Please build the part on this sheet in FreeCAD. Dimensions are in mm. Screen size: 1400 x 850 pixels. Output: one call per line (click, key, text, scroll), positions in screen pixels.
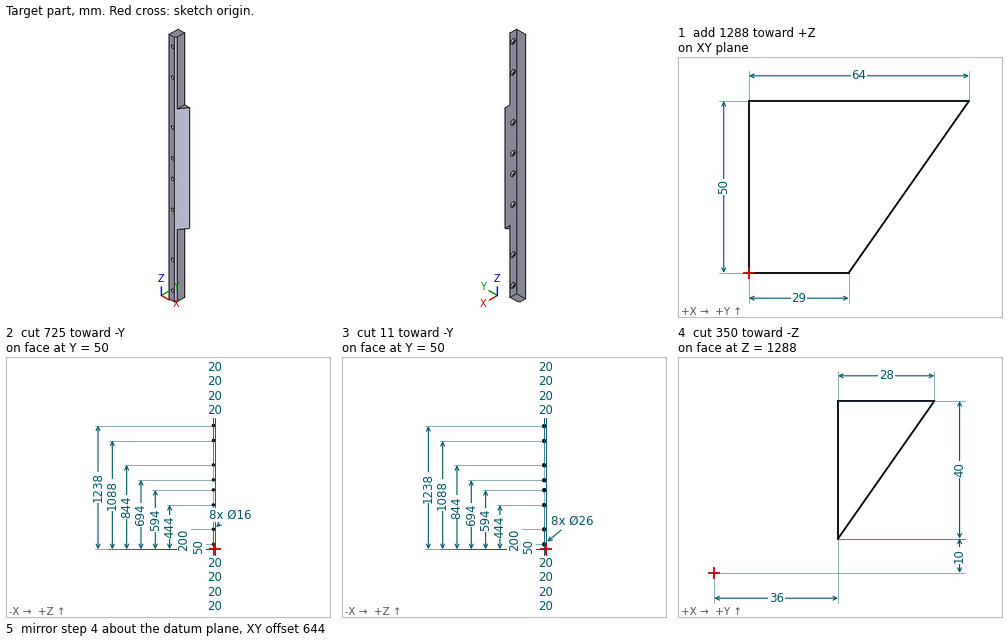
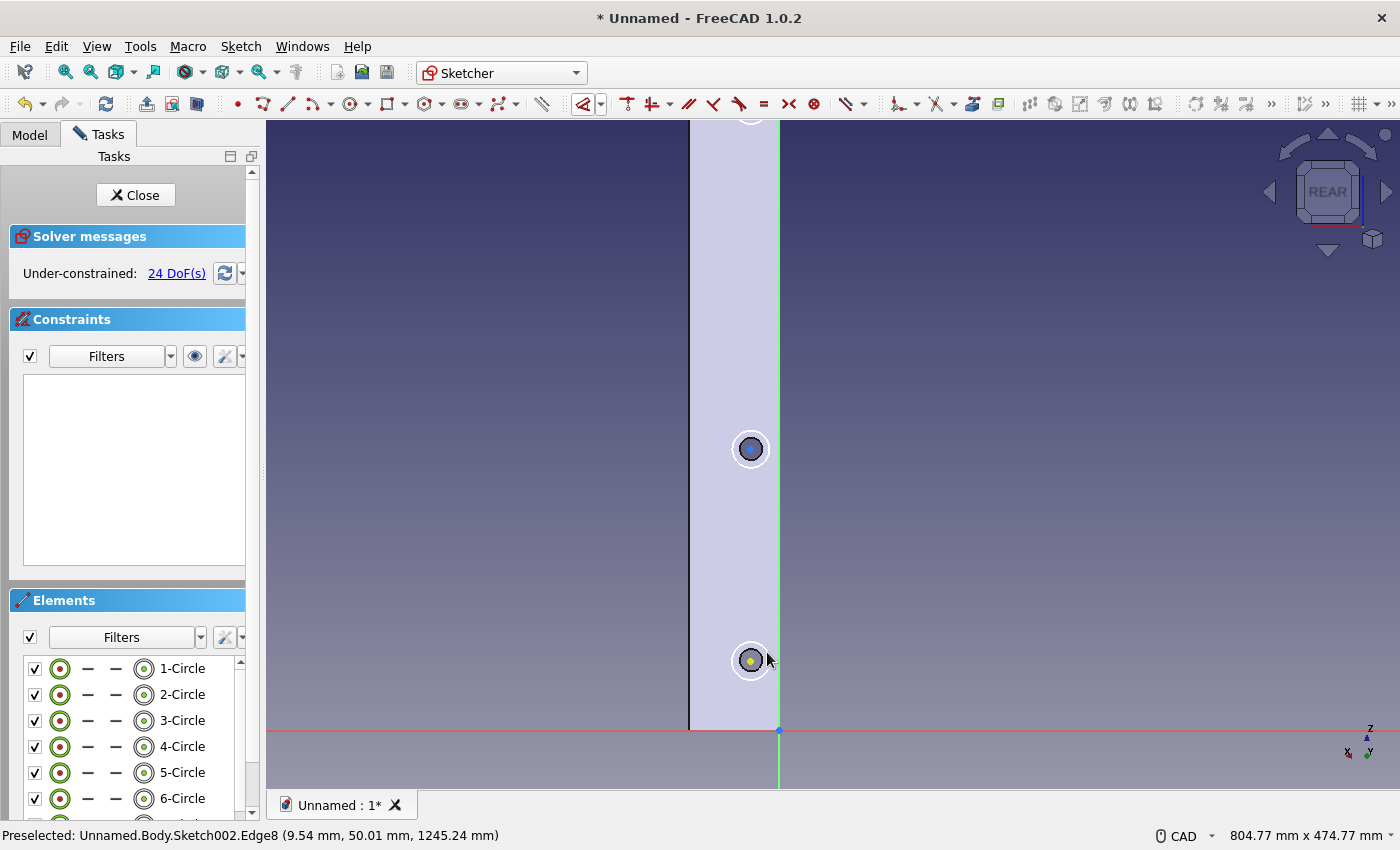
click(764, 648)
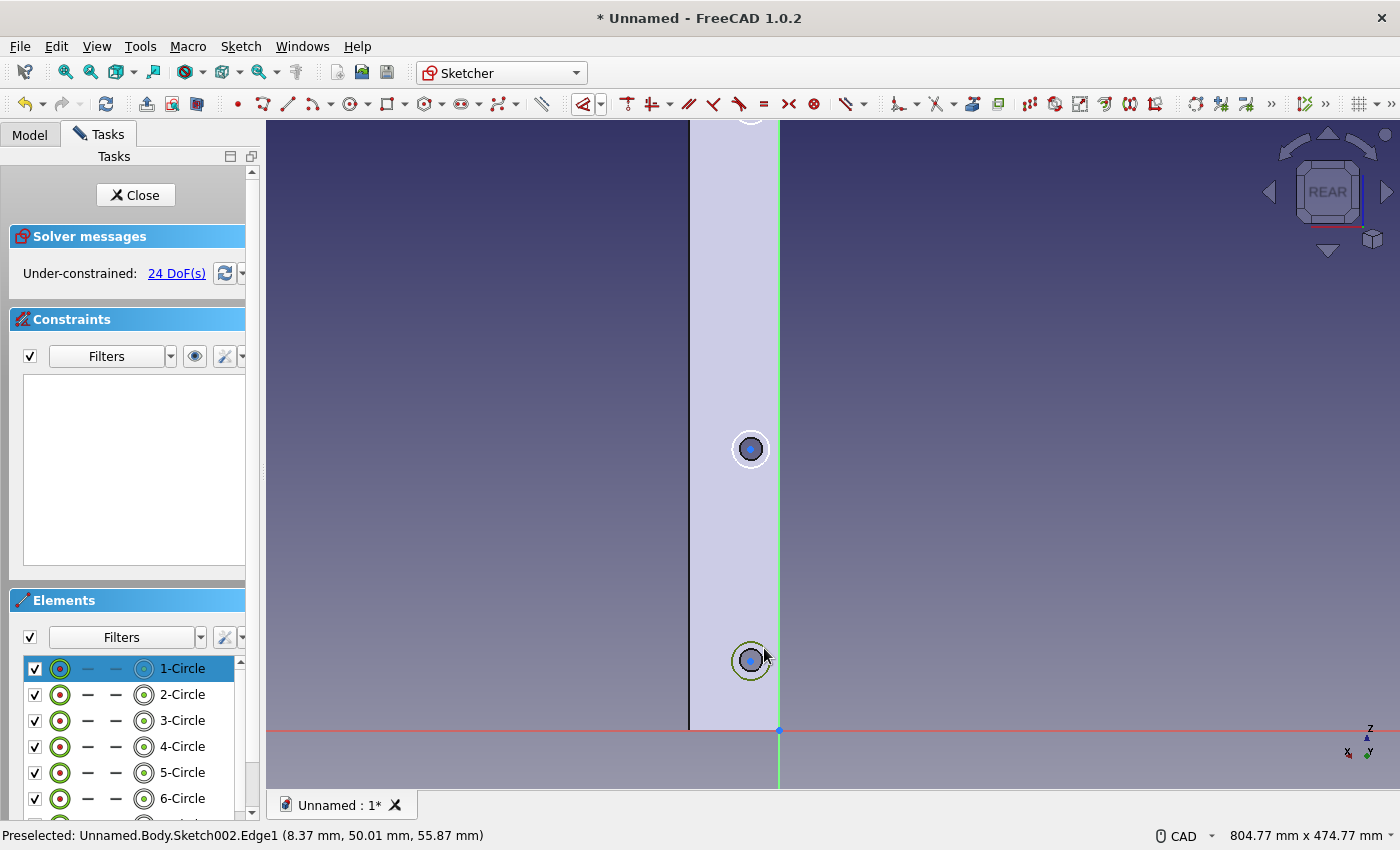
click(764, 436)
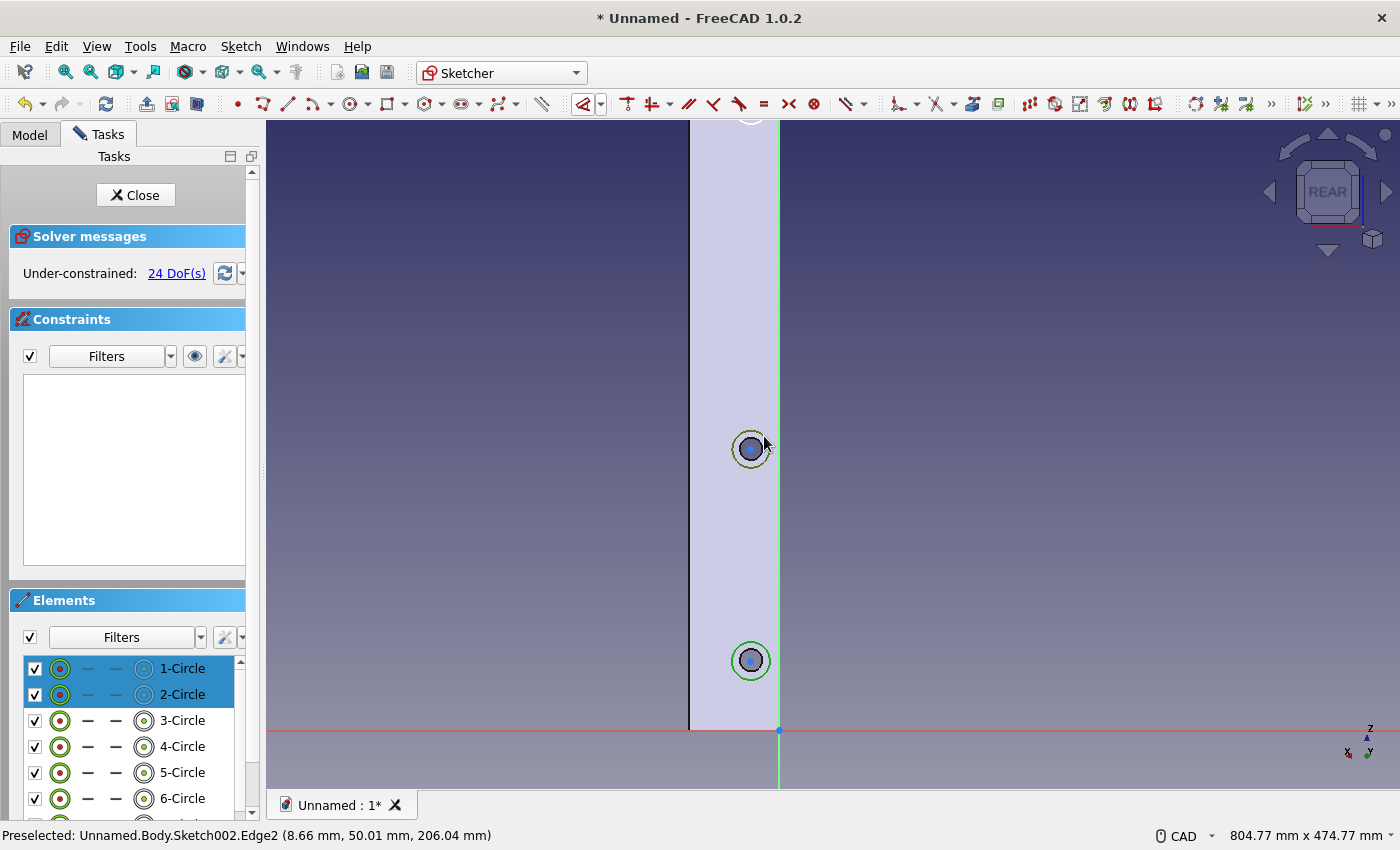
scroll(767, 653, down, 7)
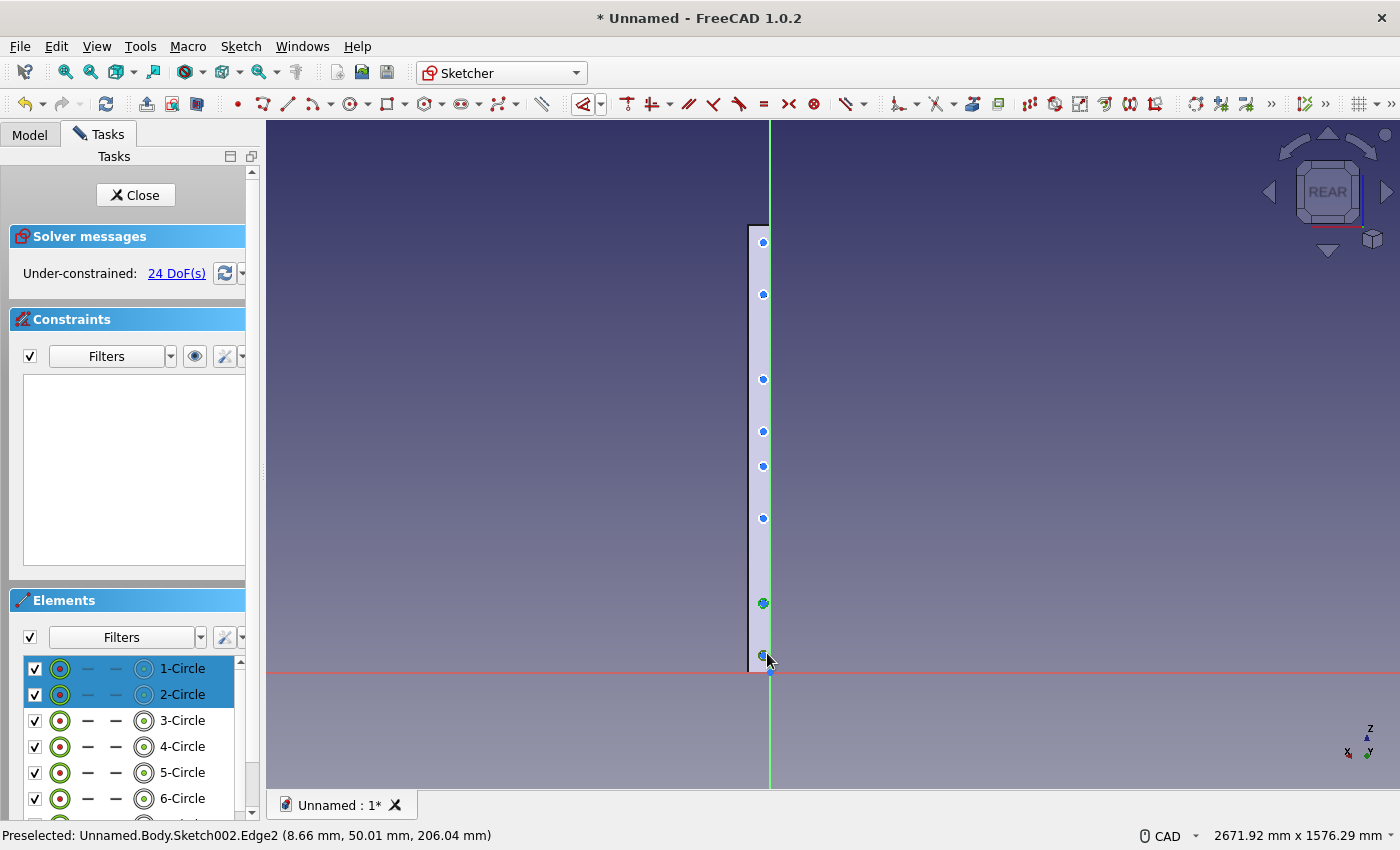
scroll(767, 515, up, 7)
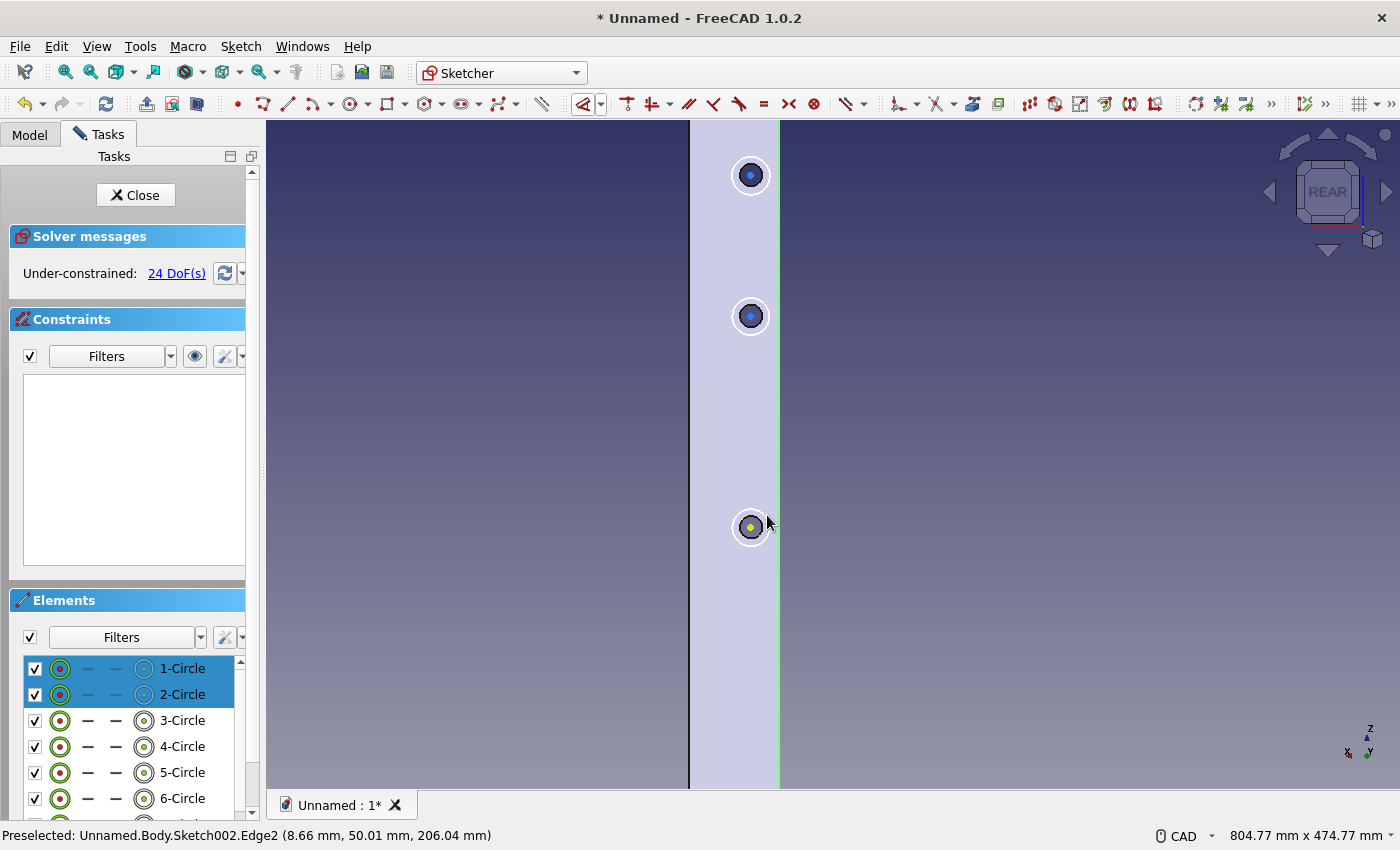
click(764, 515)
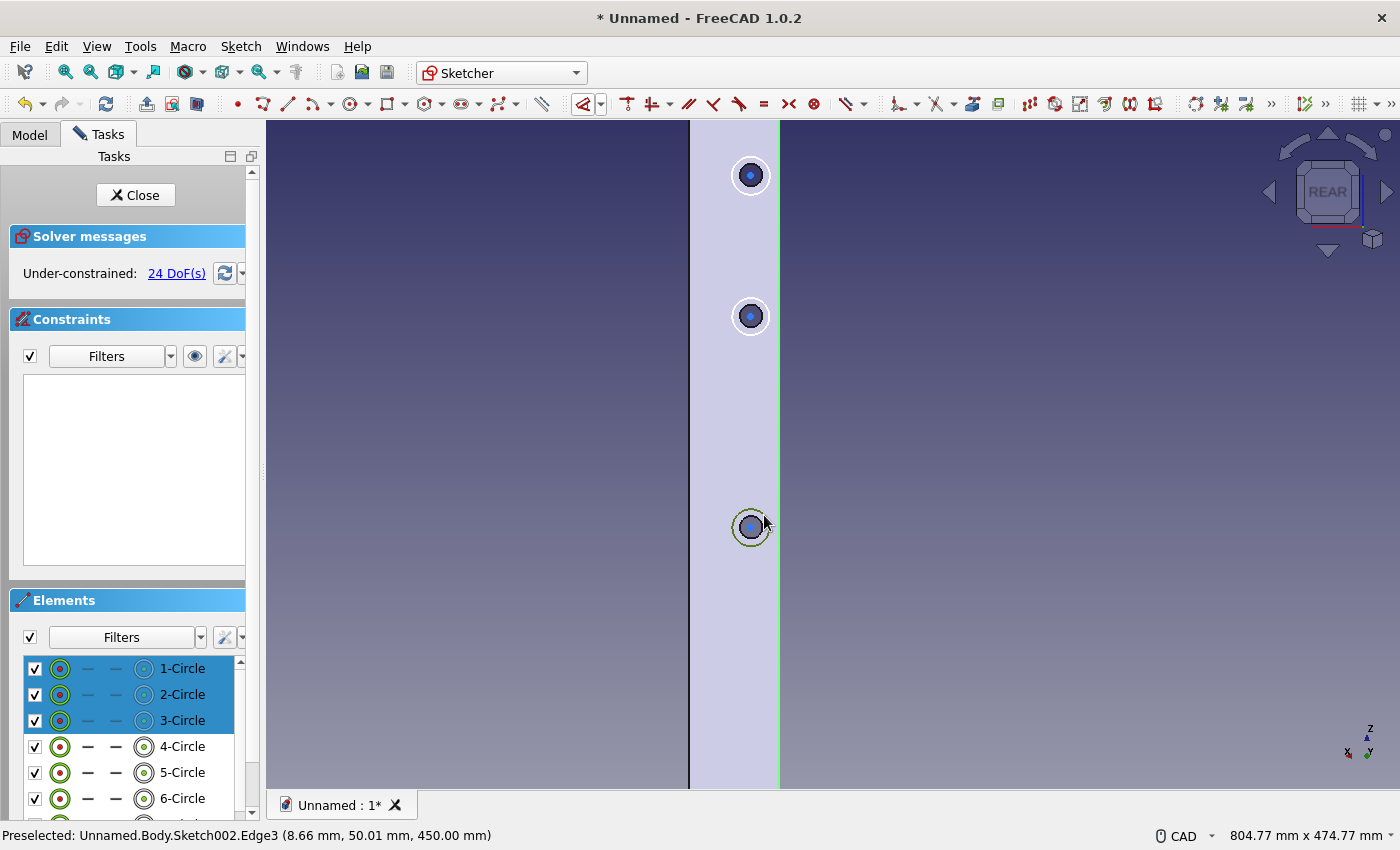
click(764, 303)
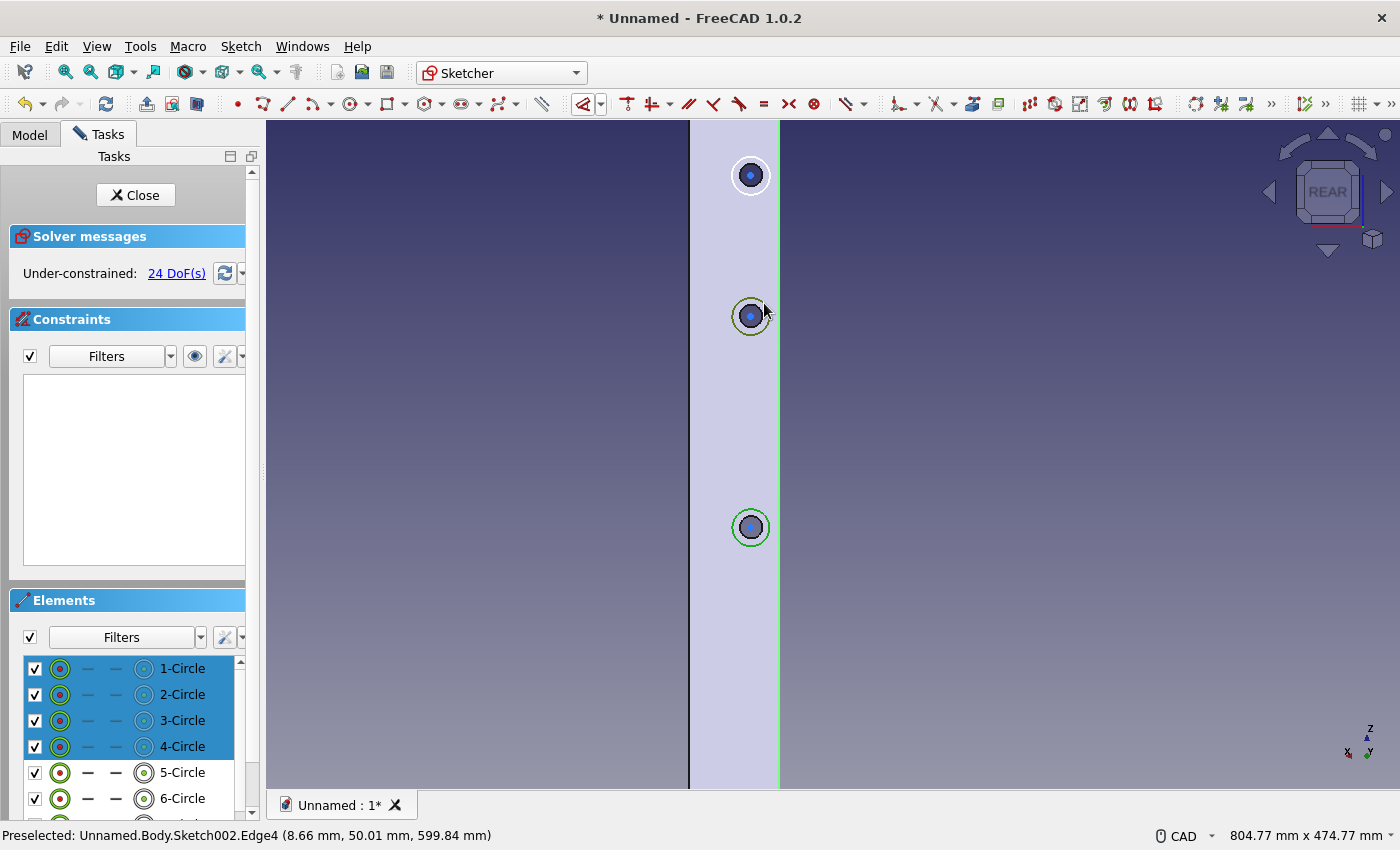
click(764, 162)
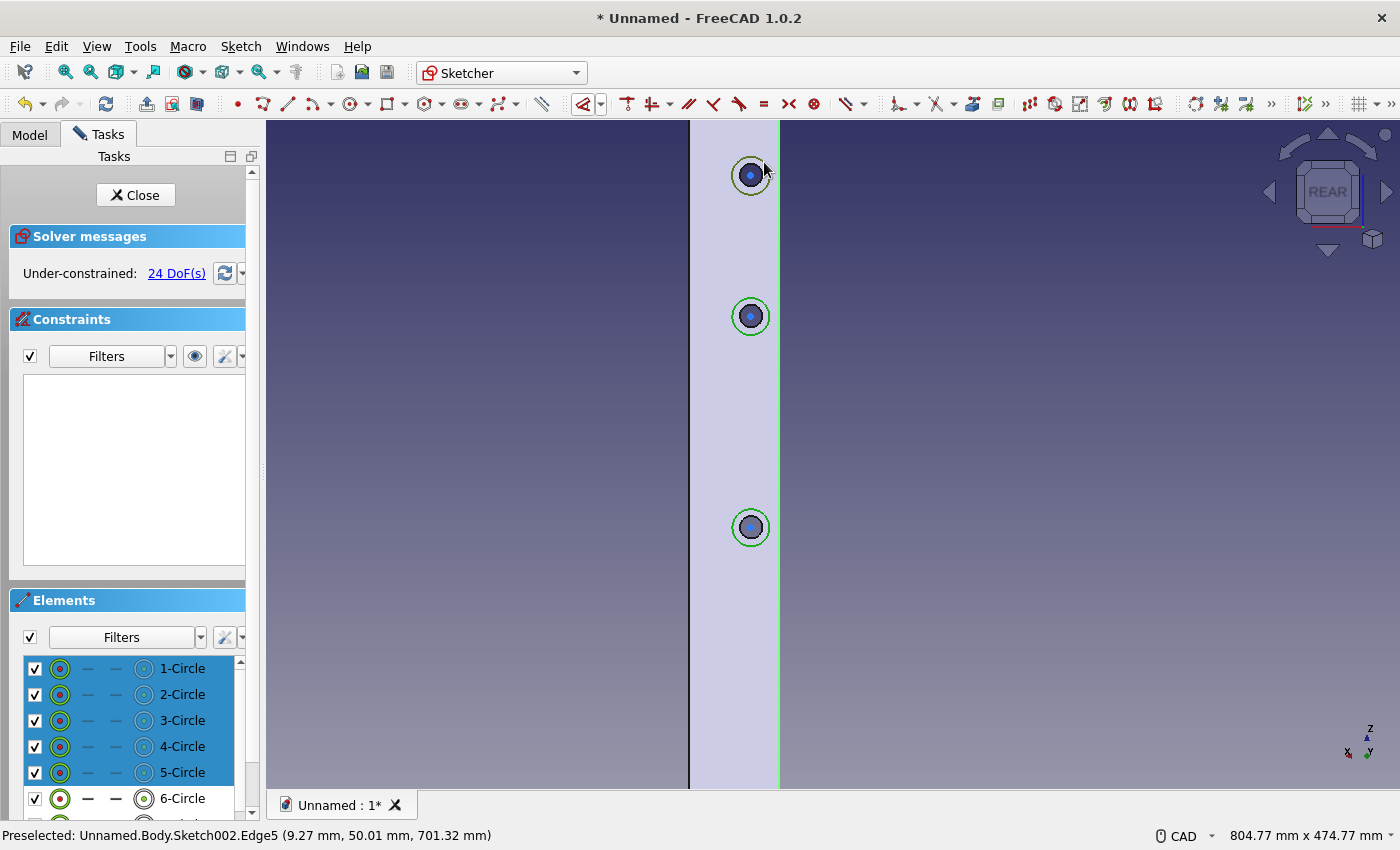
scroll(767, 514, down, 7)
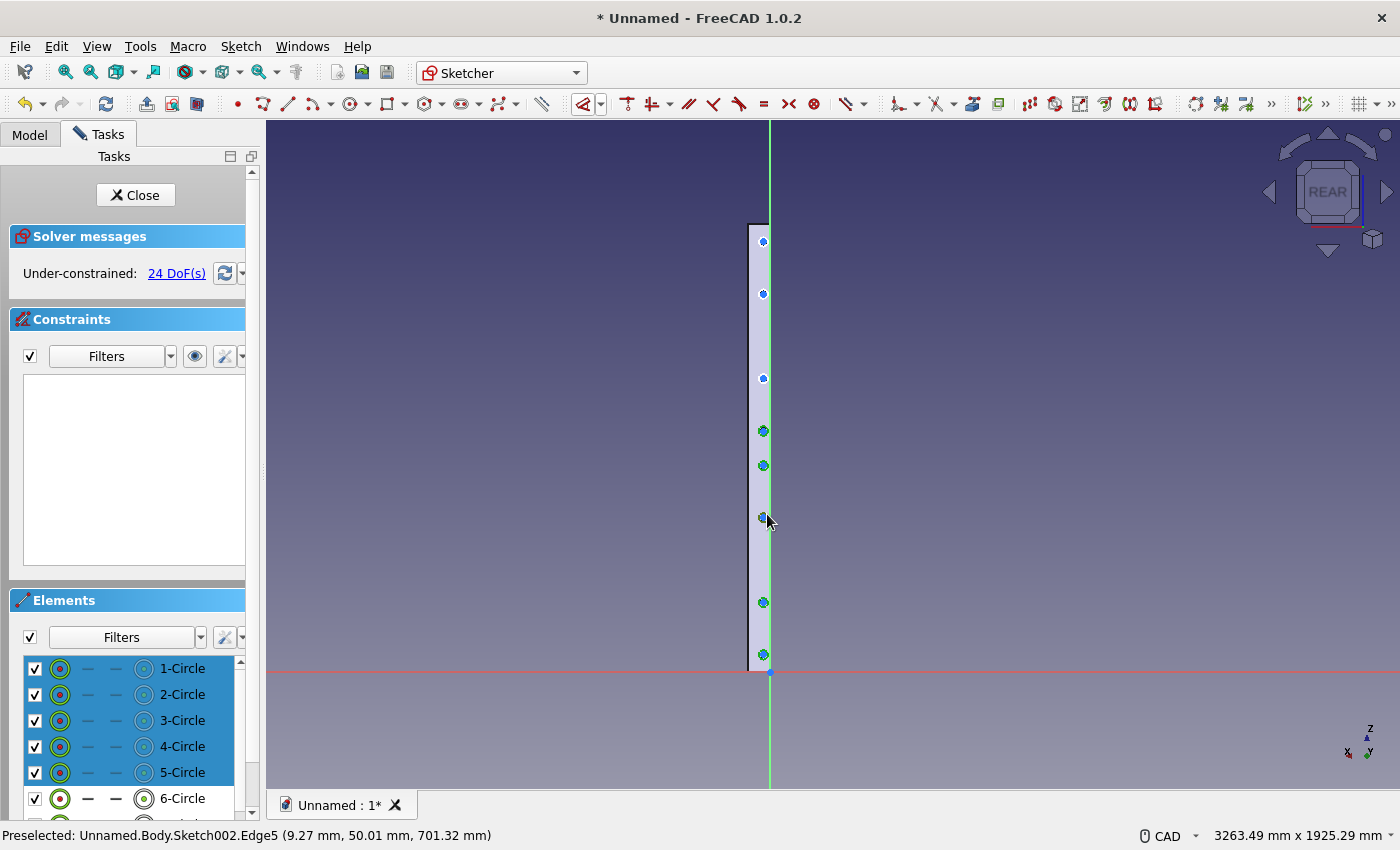
scroll(767, 376, up, 7)